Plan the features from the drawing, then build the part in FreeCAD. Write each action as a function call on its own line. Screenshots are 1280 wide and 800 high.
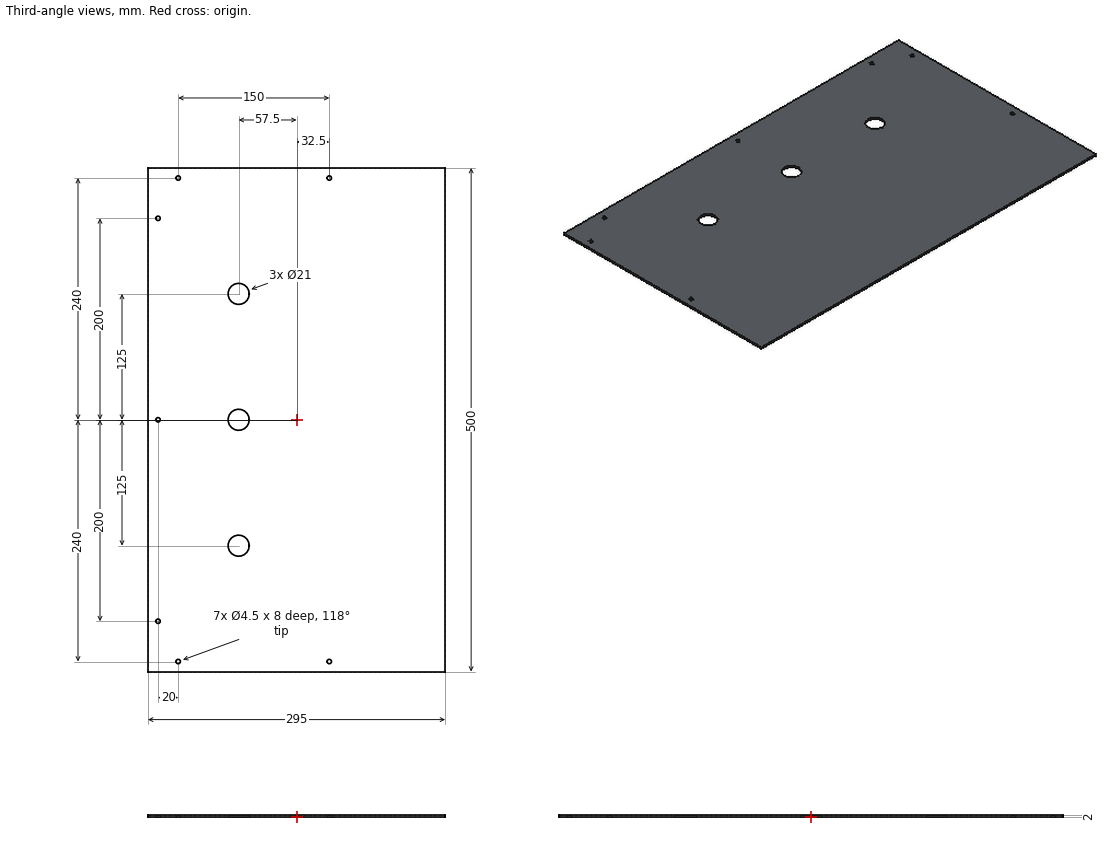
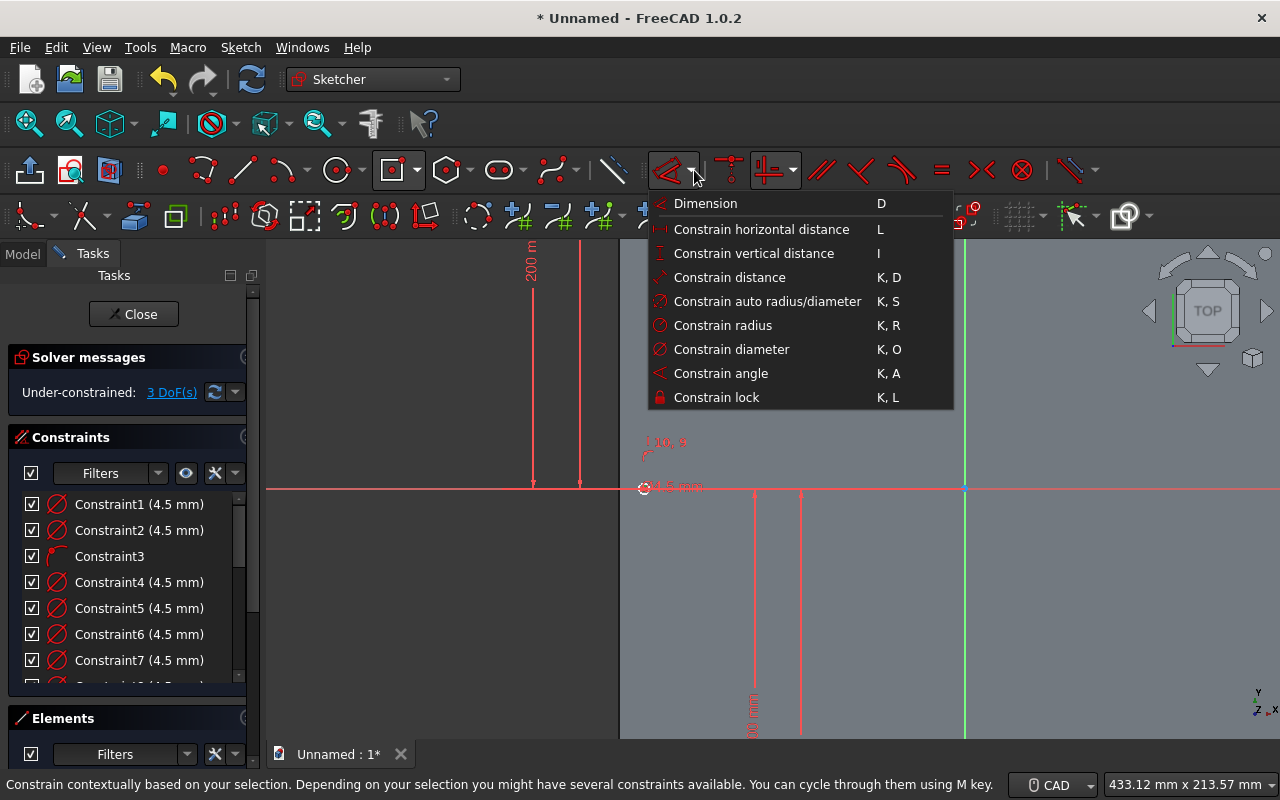
click(801, 229)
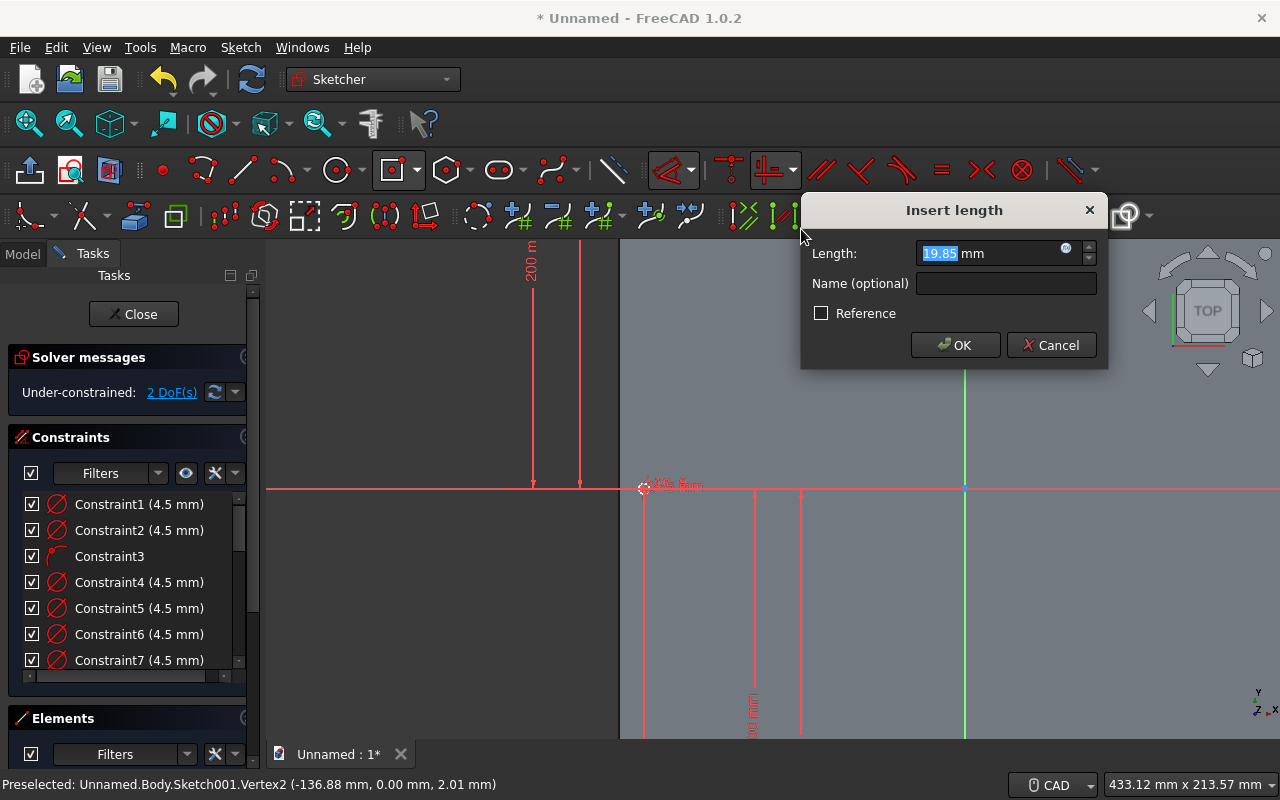
text(20)
key(Return)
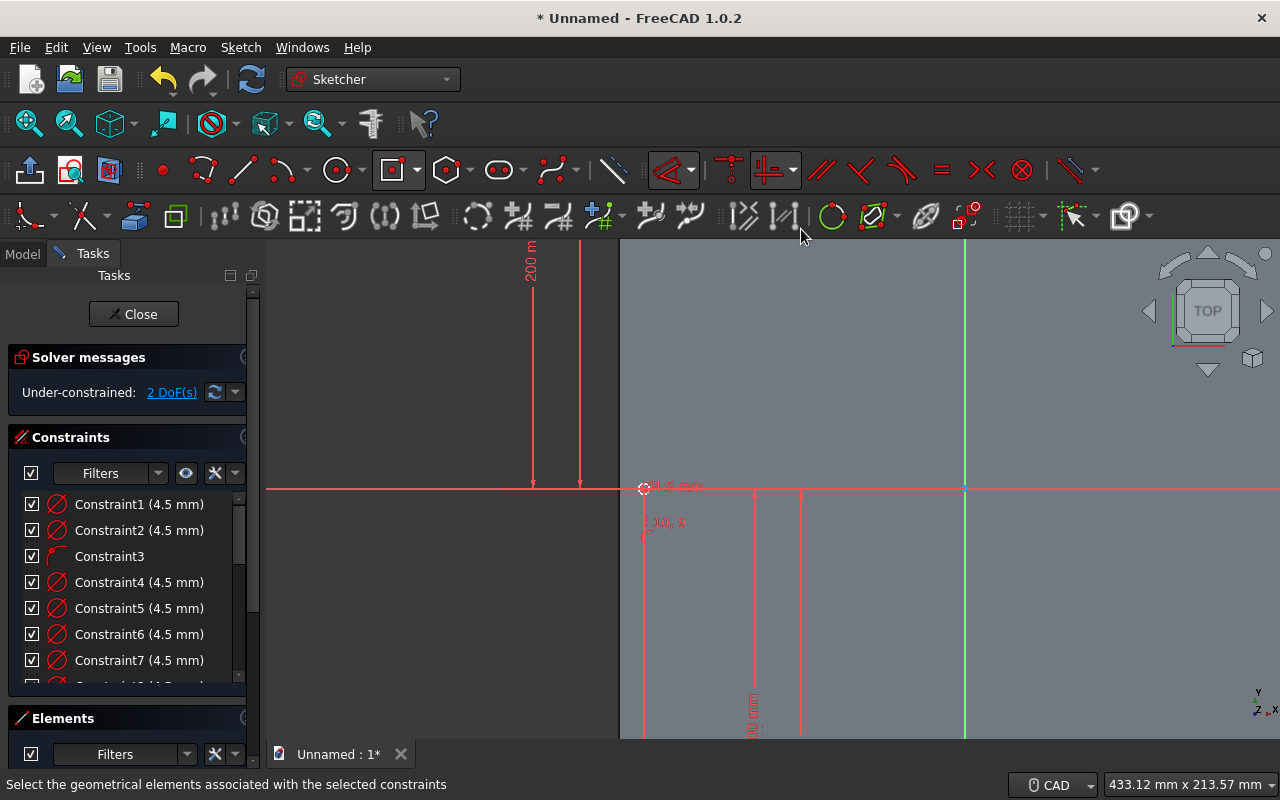
scroll(645, 489, down, 6)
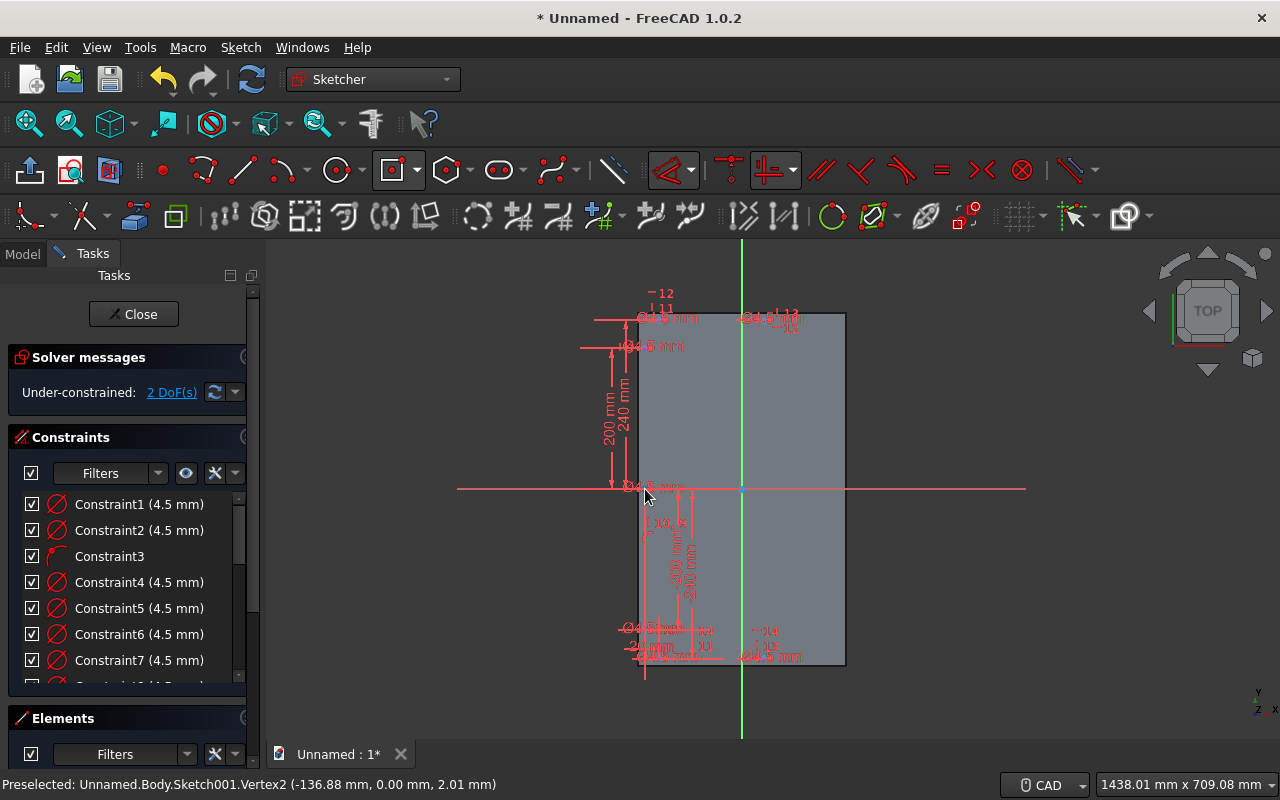
scroll(764, 320, up, 3)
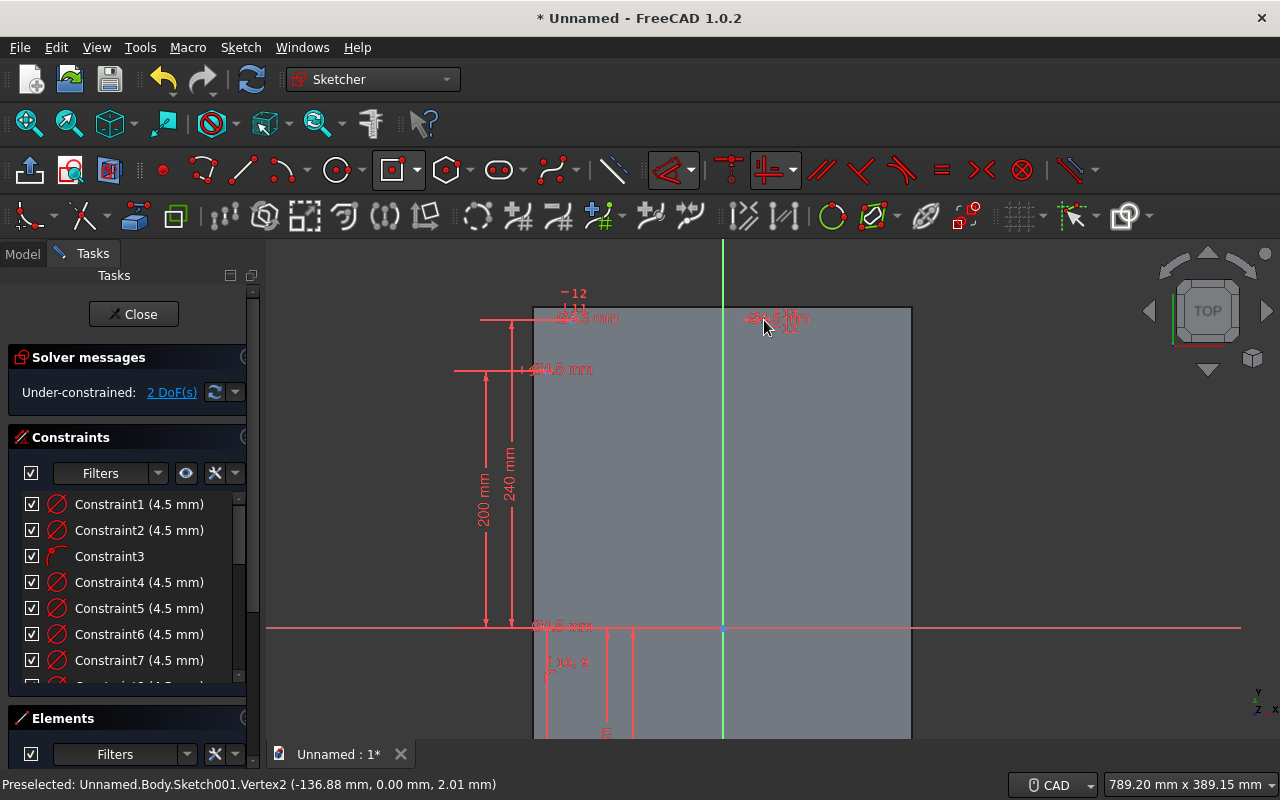
click(764, 320)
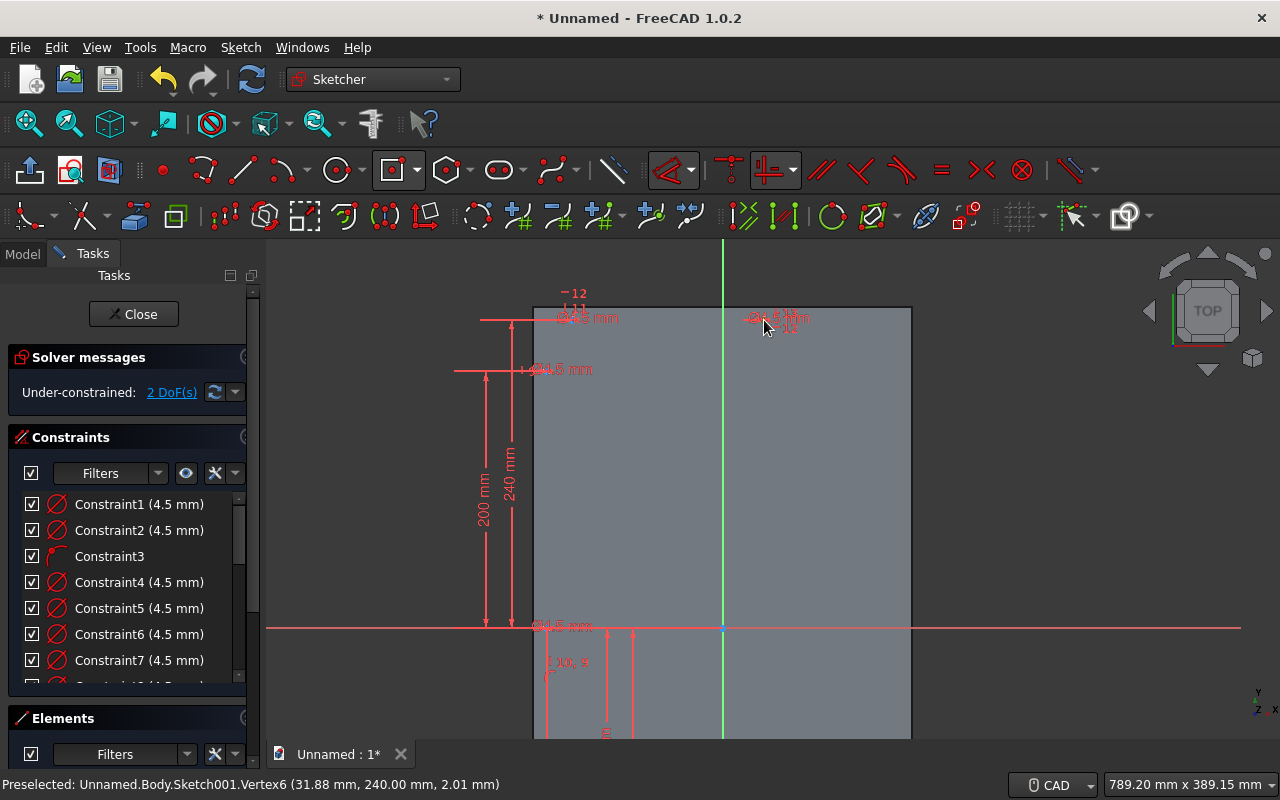
key(l)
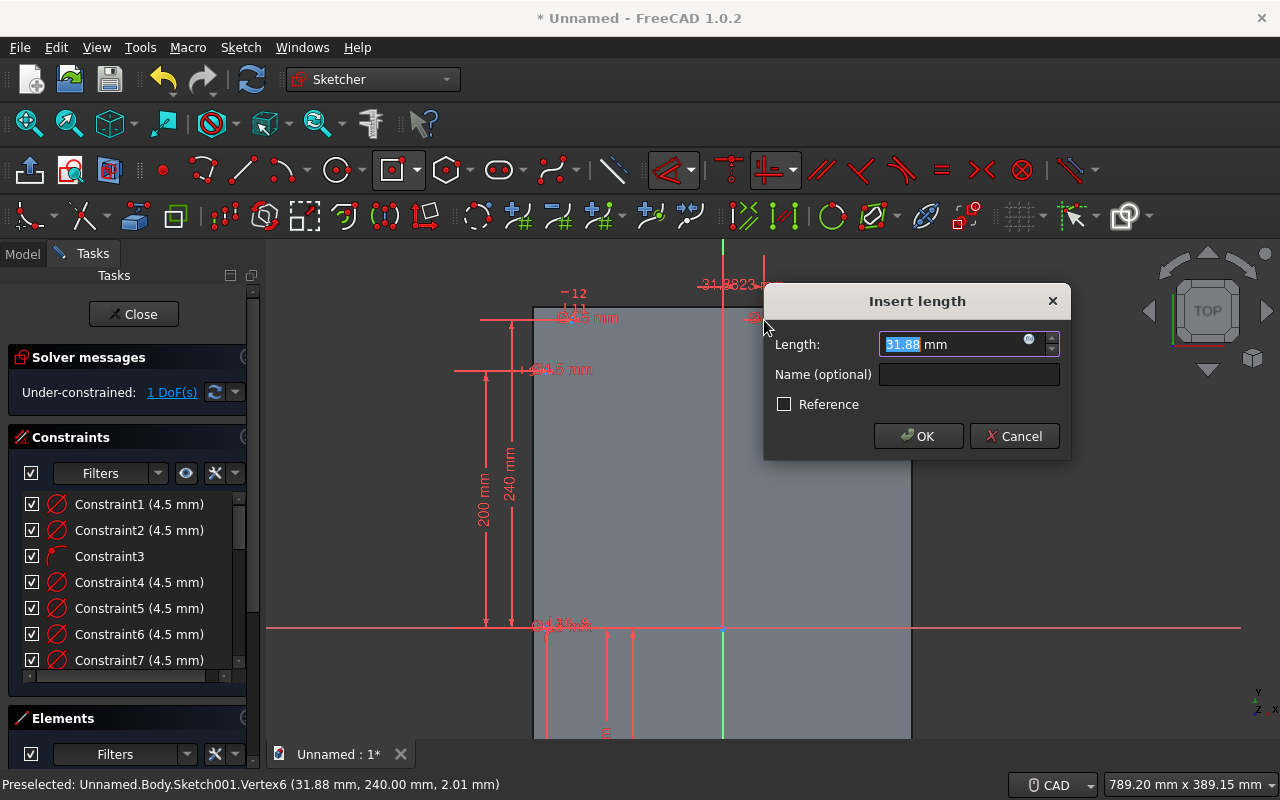
text(32.5)
key(Return)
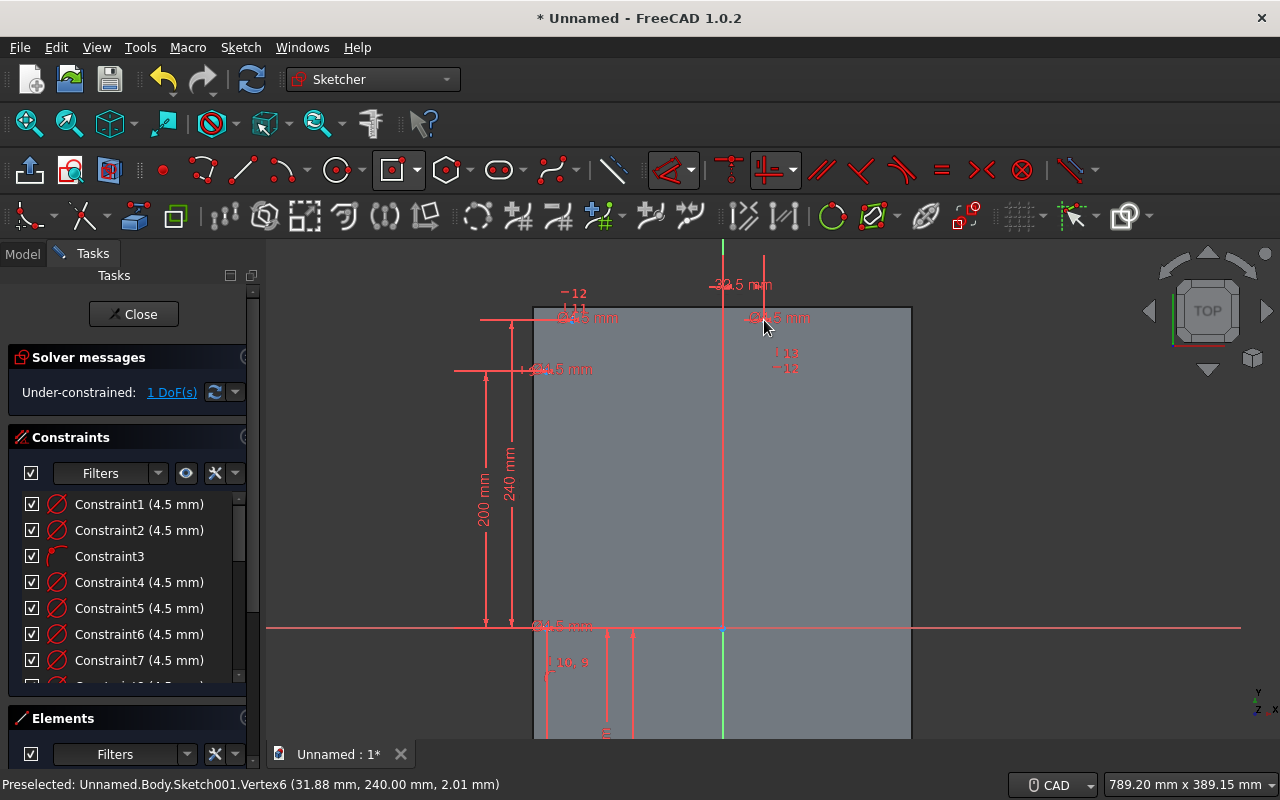
click(572, 320)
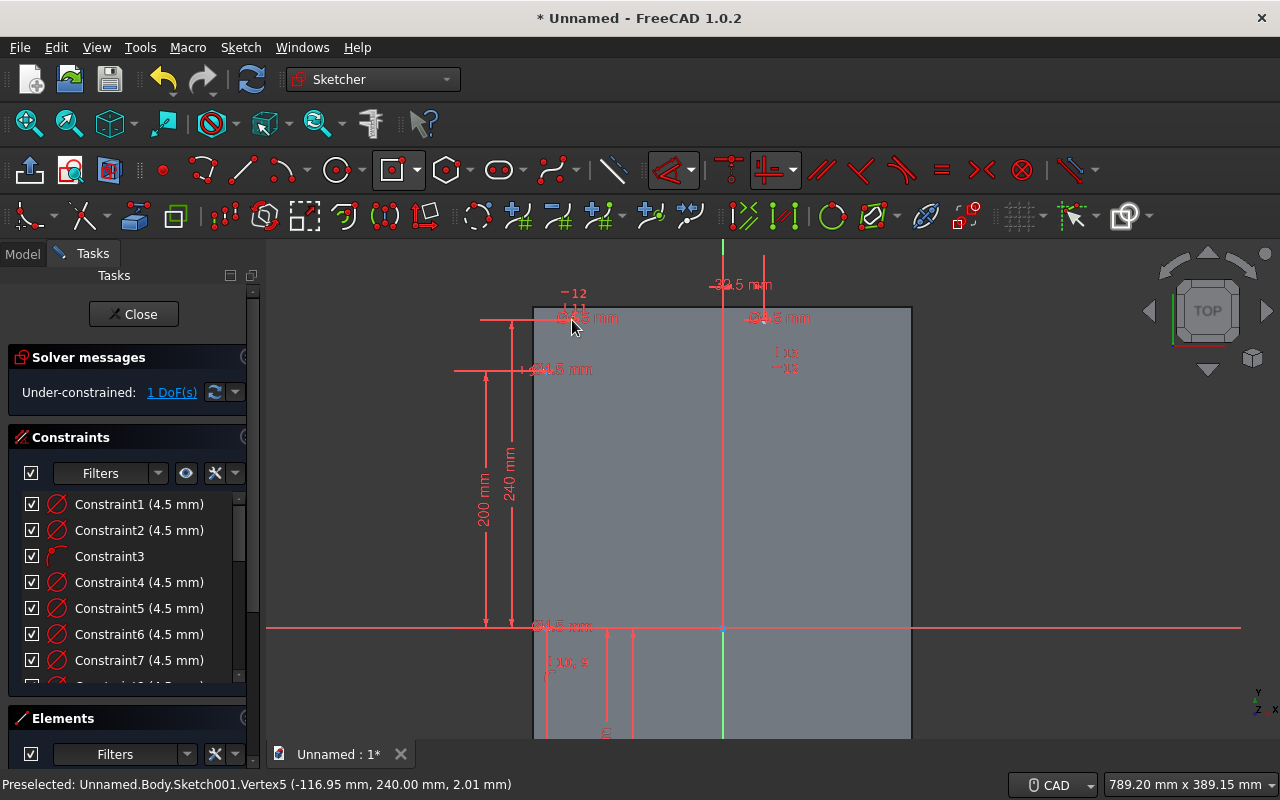
click(764, 320)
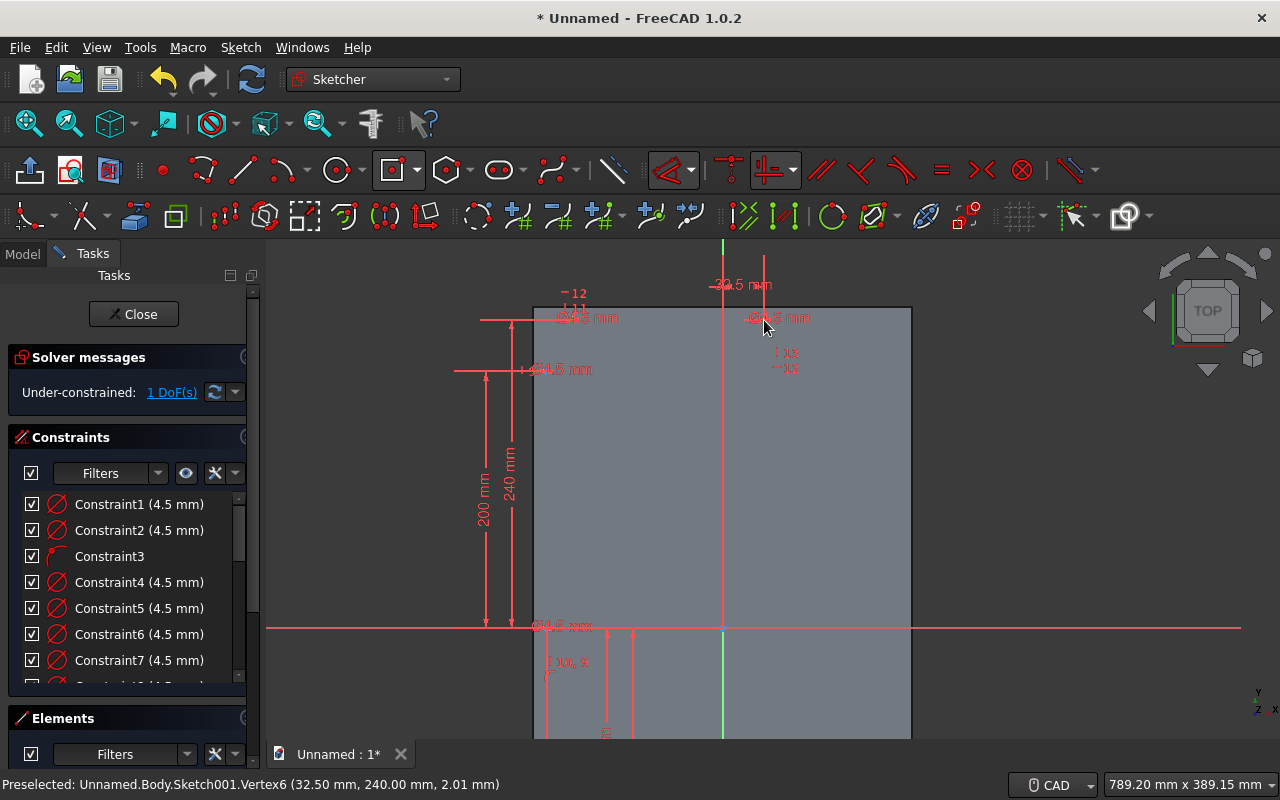
click(694, 170)